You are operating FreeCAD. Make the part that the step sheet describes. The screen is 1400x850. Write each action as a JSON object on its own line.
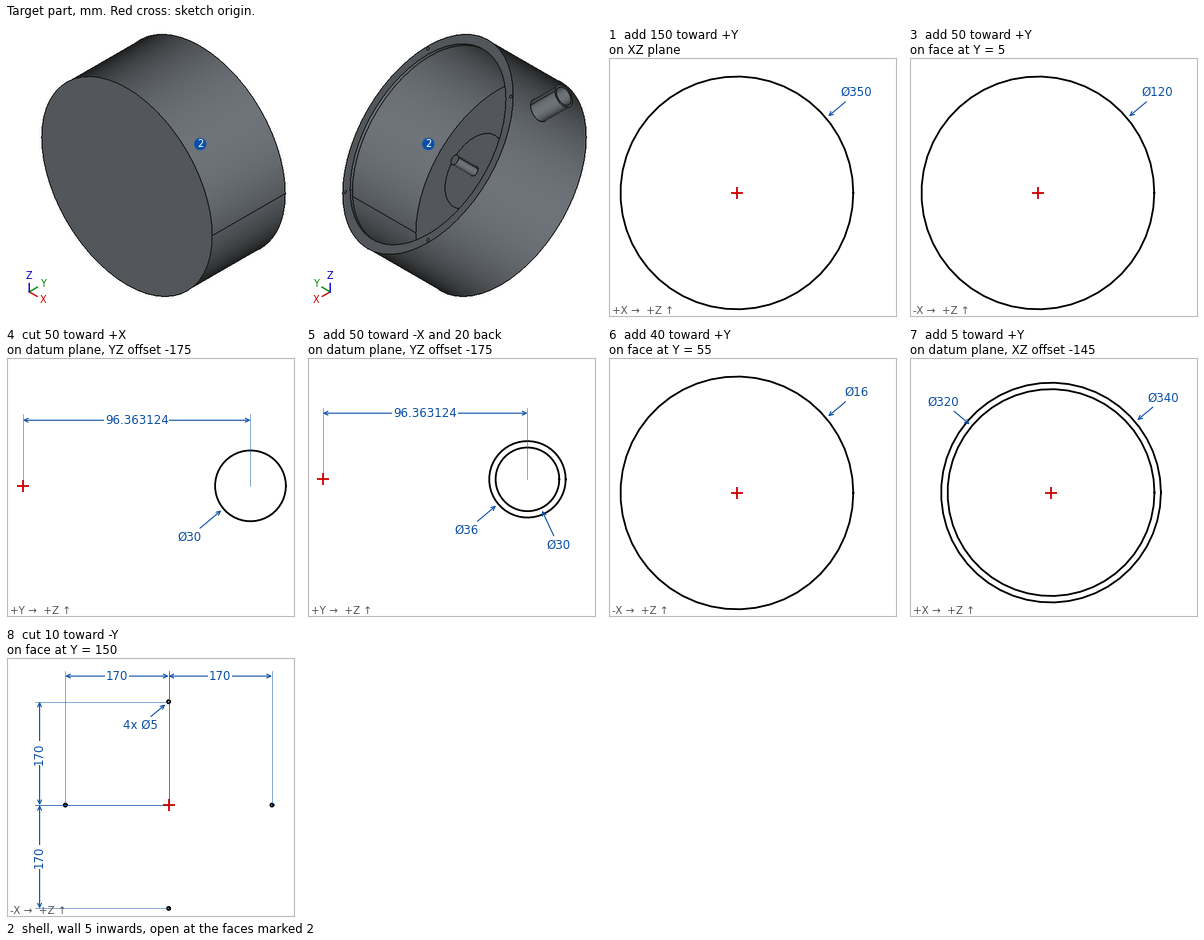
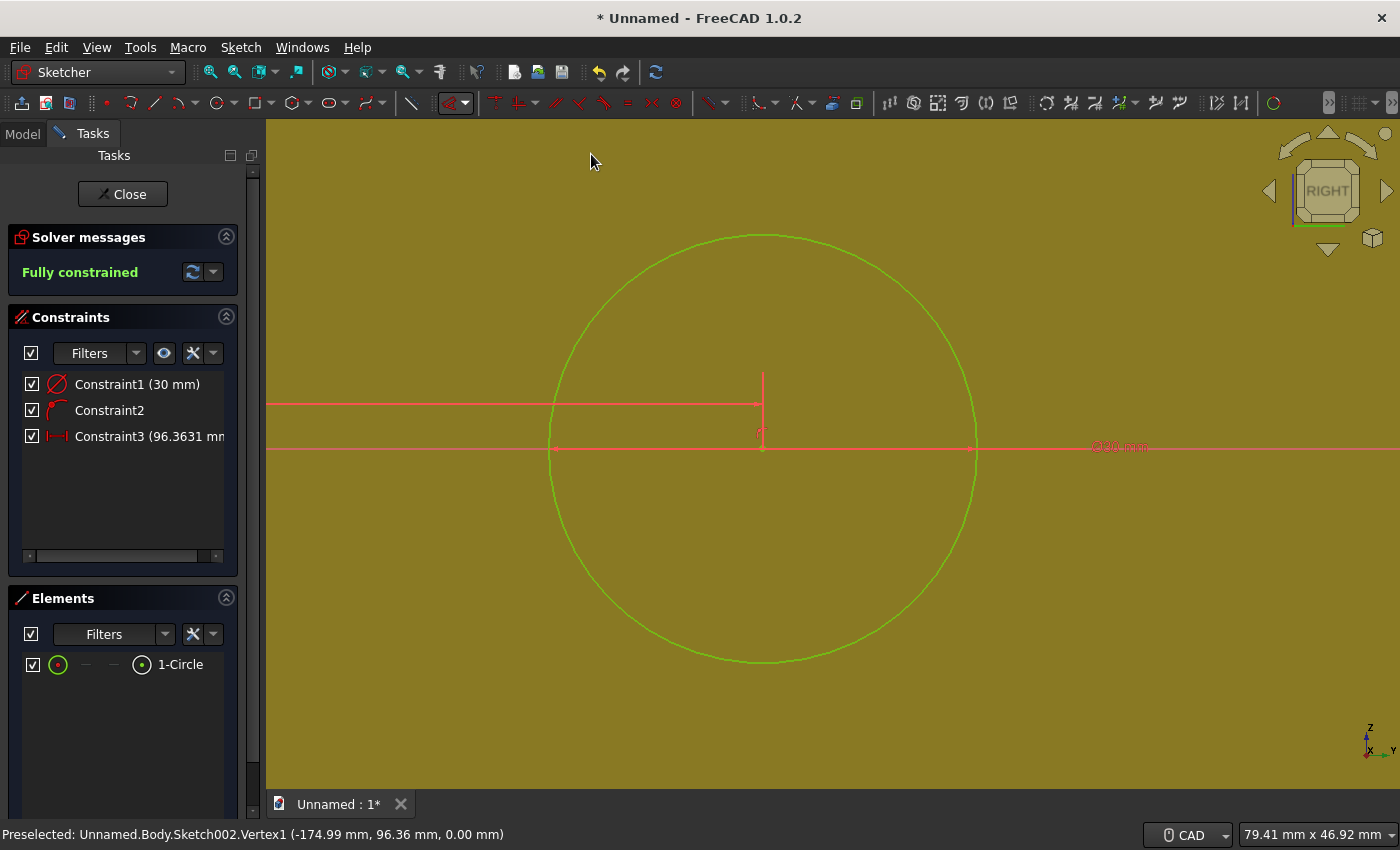
{"action": "left_click", "coordinate": [123, 194]}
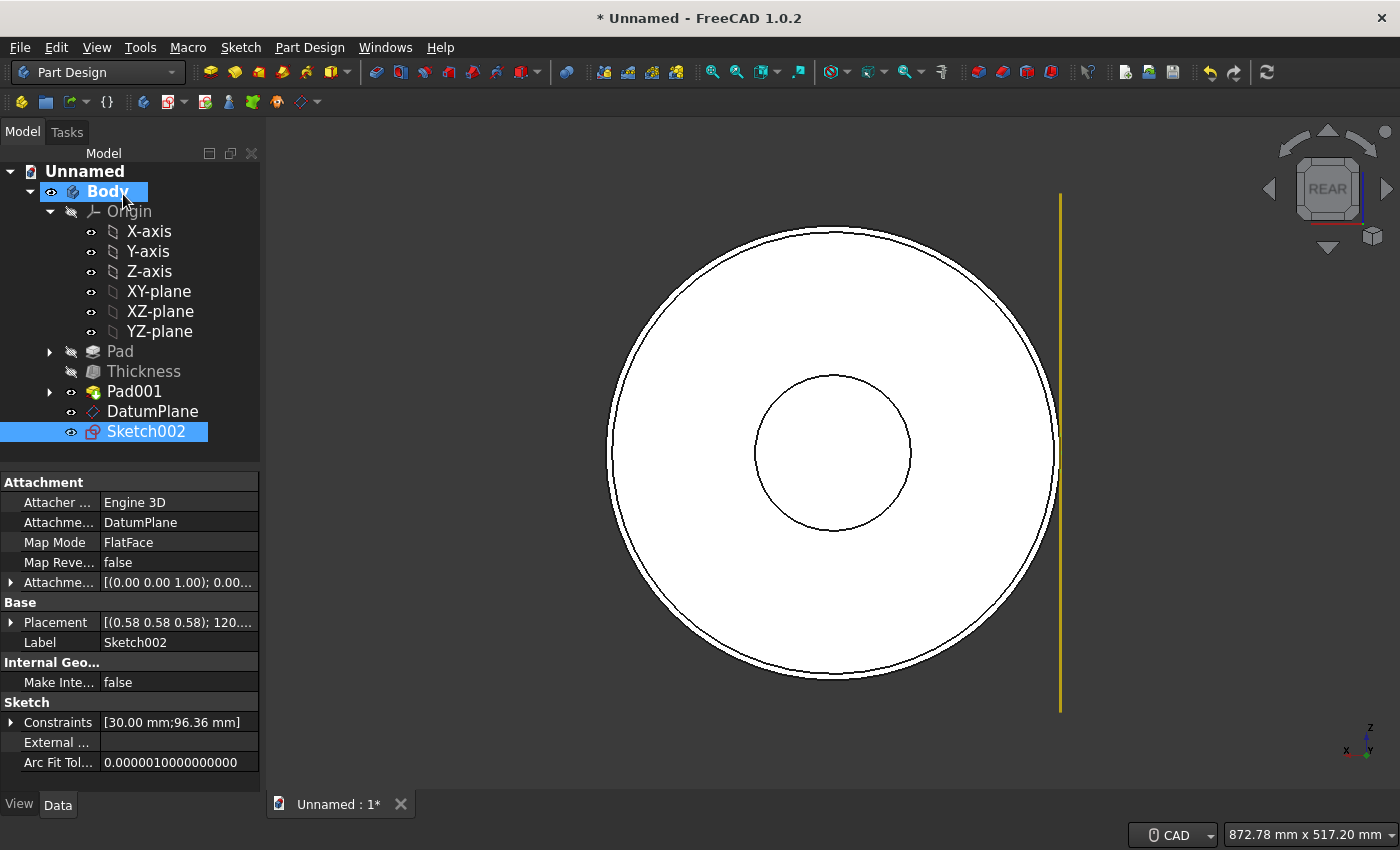
{"action": "left_click", "coordinate": [378, 72]}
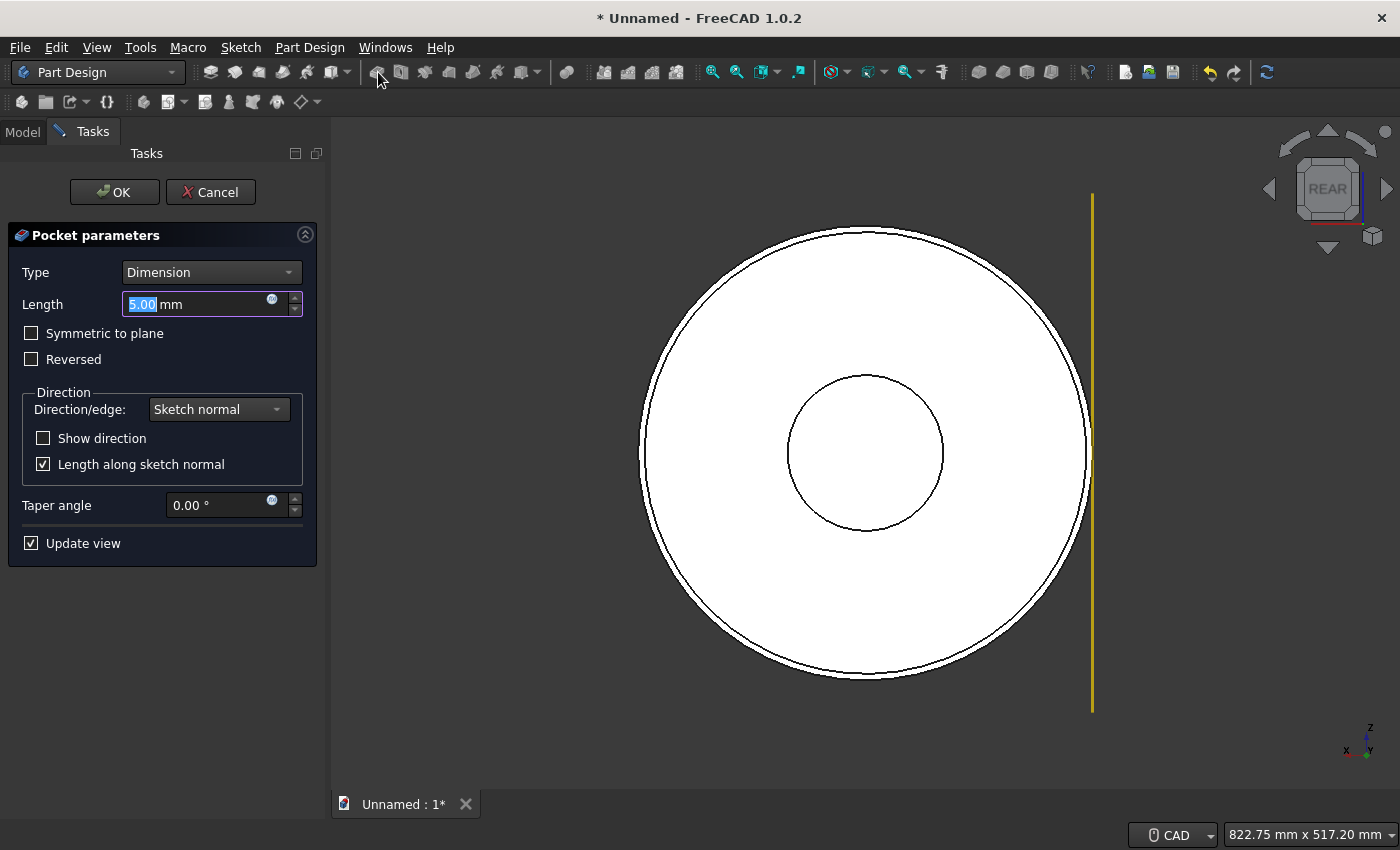
{"action": "type", "text": "50"}
{"action": "key", "text": "Tab"}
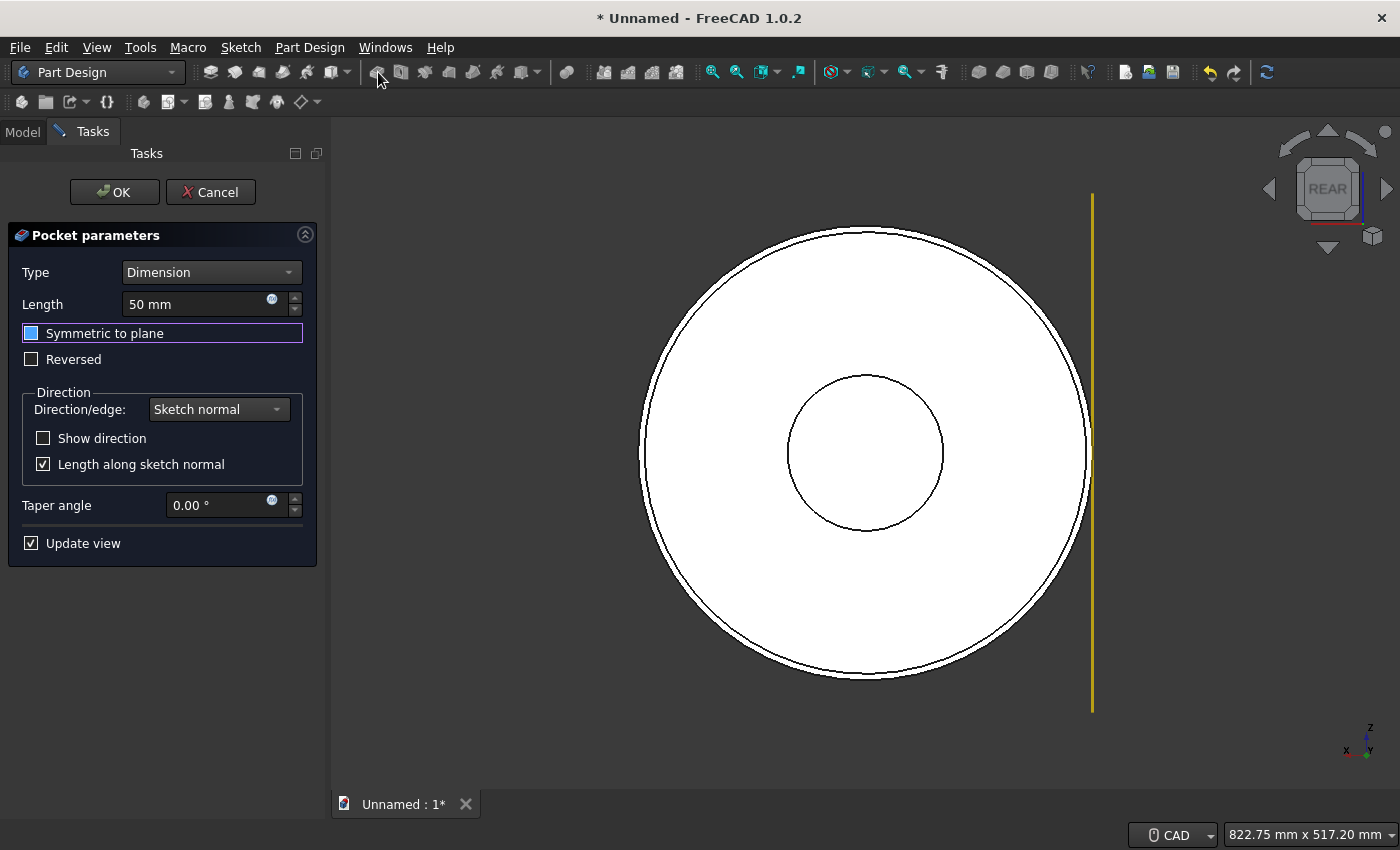
{"action": "left_click", "coordinate": [30, 359]}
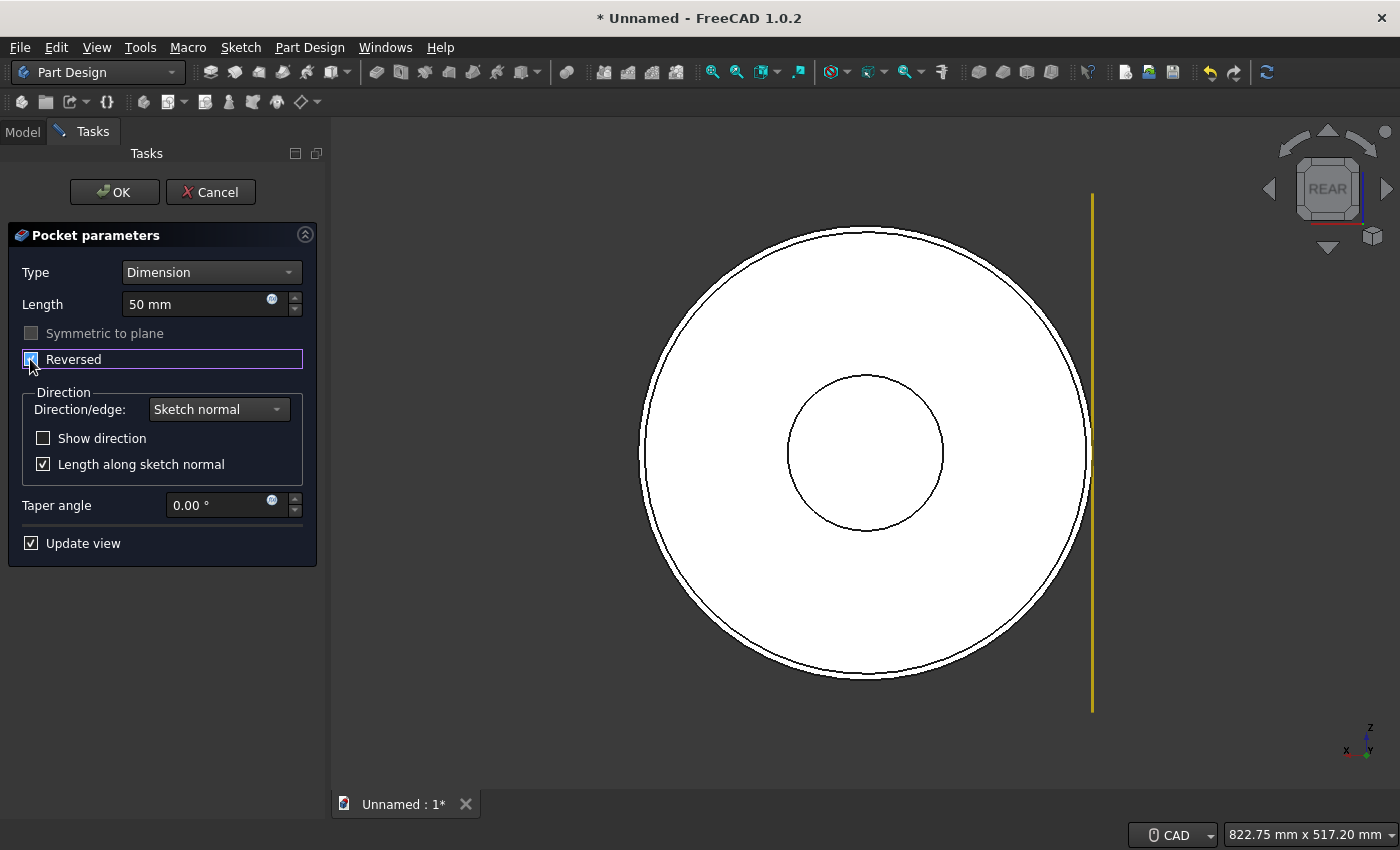
{"action": "left_click", "coordinate": [115, 192]}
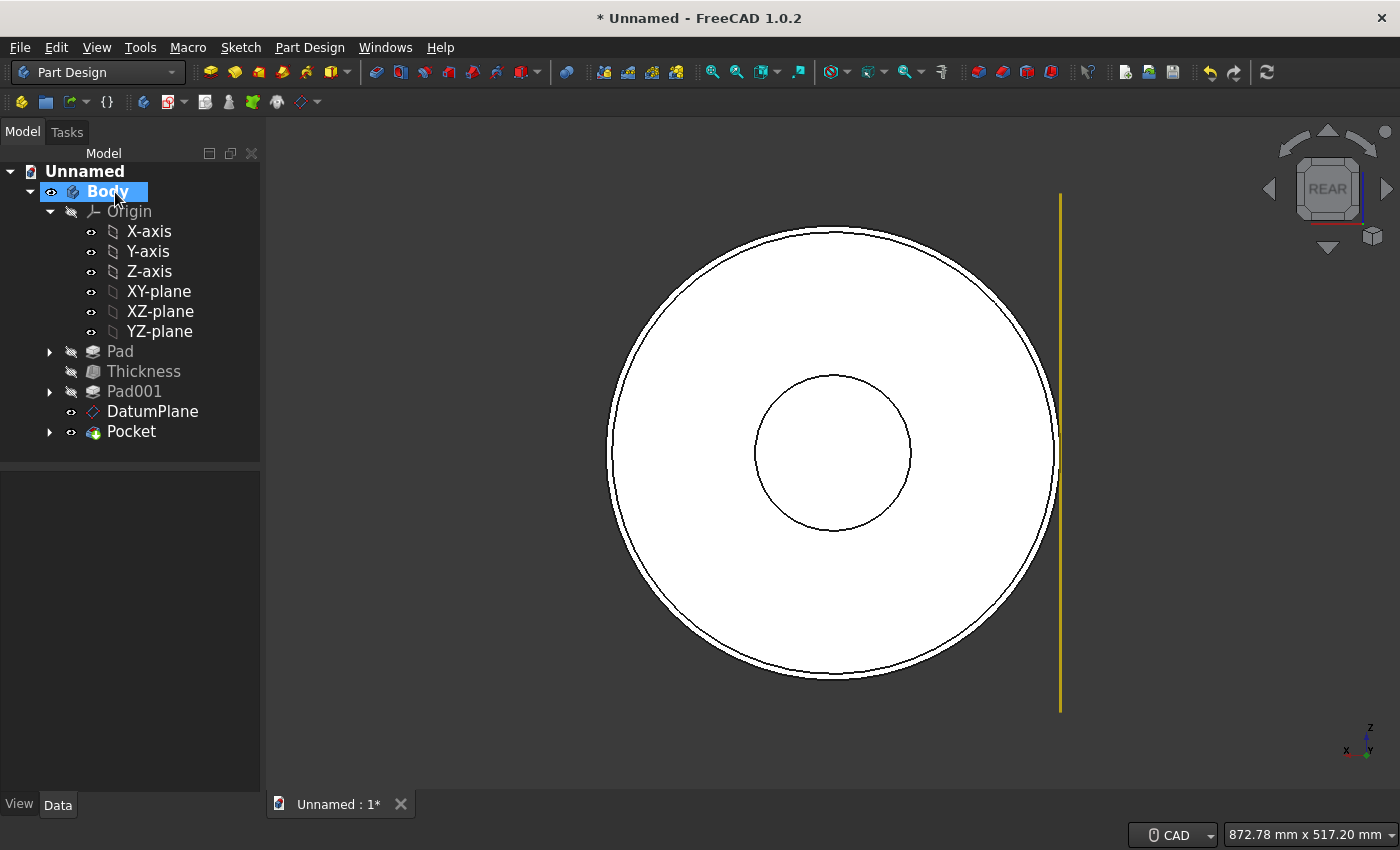
{"action": "left_click", "coordinate": [116, 412]}
{"action": "key", "text": "space"}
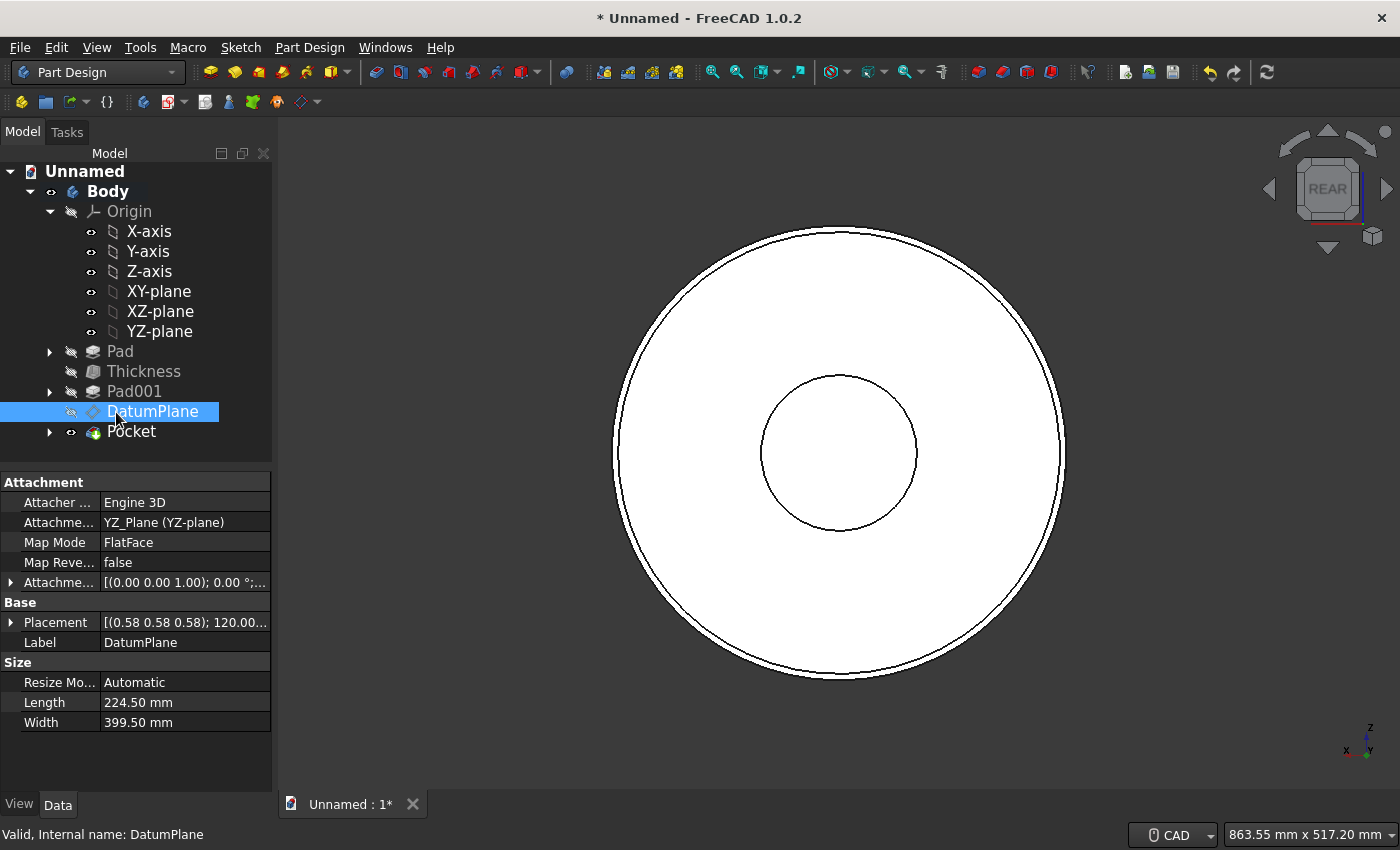
{"action": "left_click", "coordinate": [136, 332]}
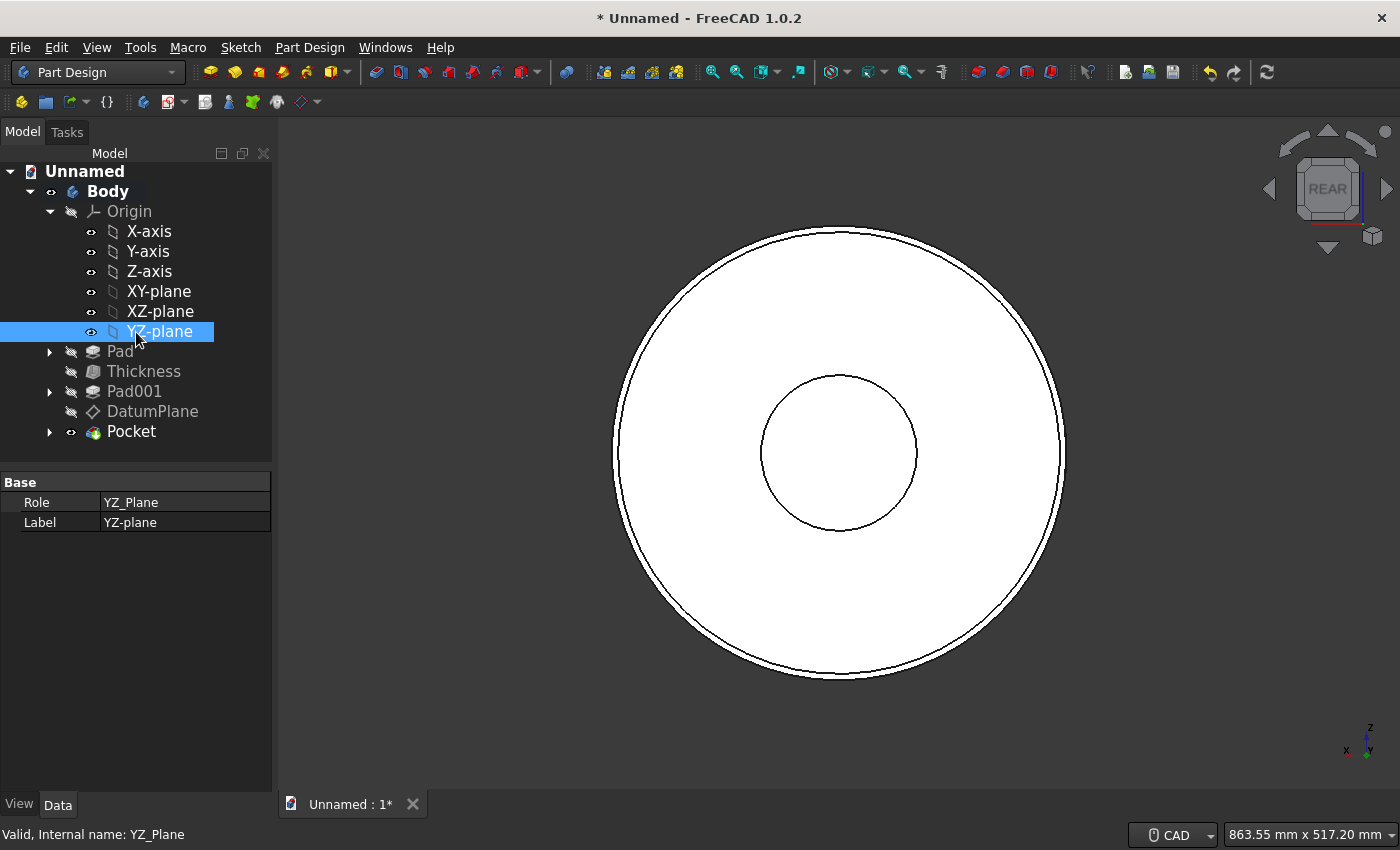
{"action": "left_click", "coordinate": [302, 102]}